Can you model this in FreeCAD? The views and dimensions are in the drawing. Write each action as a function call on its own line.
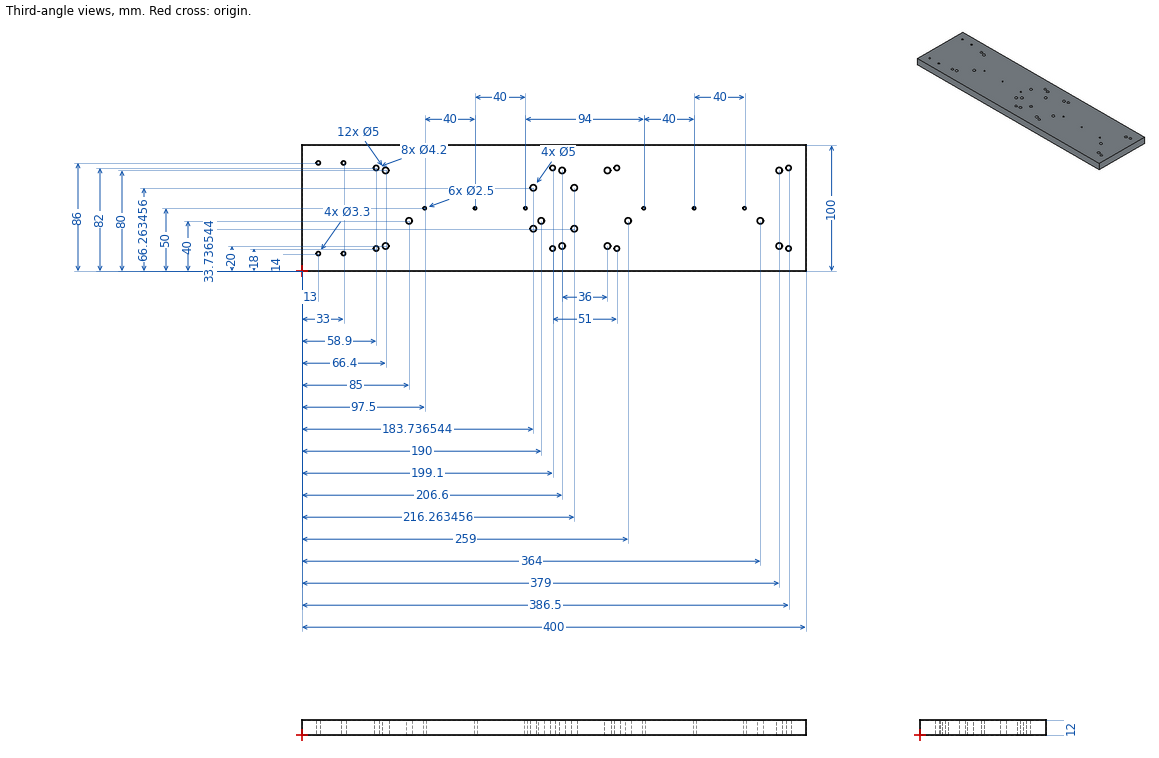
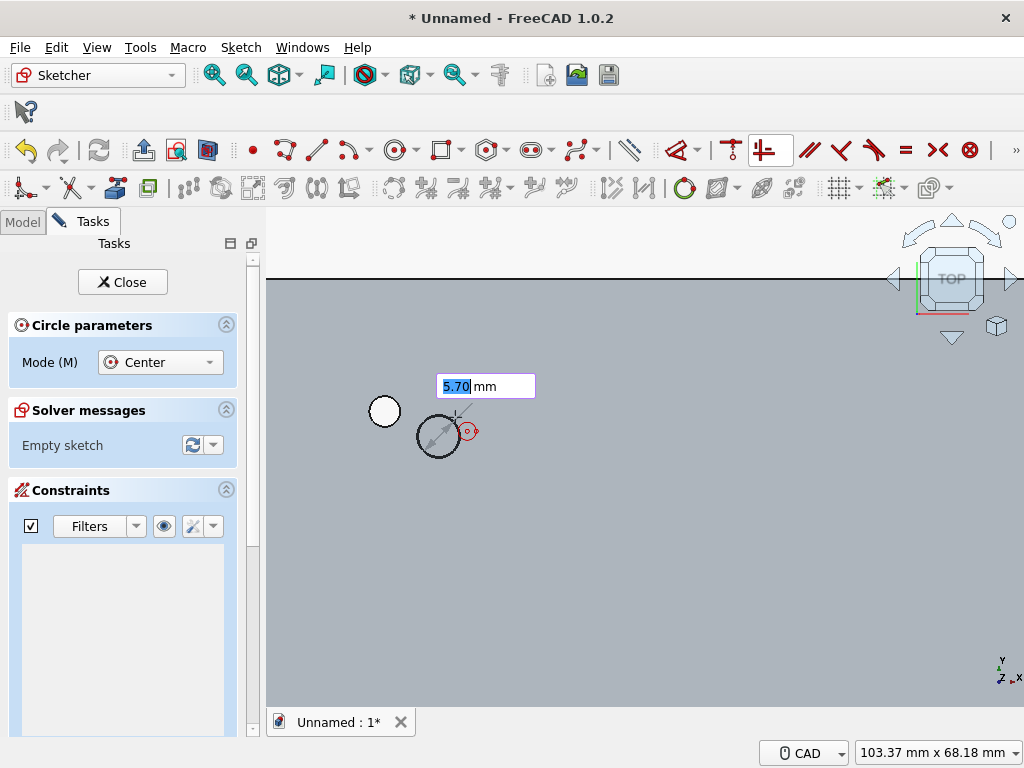
click(453, 413)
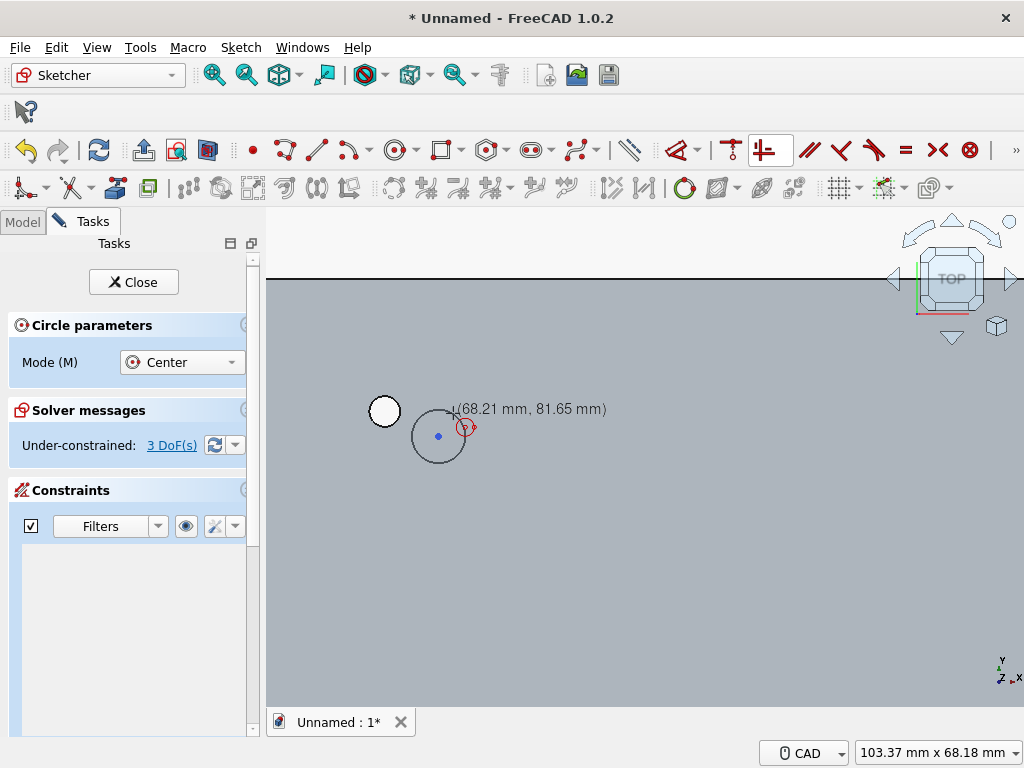
scroll(455, 417, down, 10)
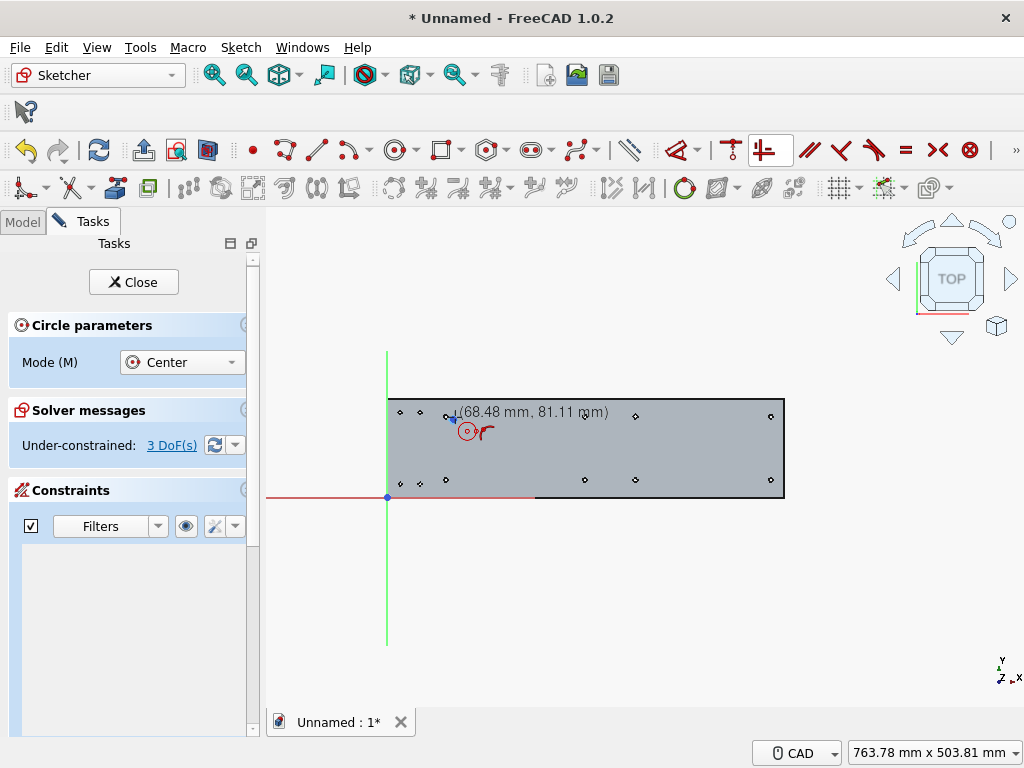
scroll(453, 478, up, 12)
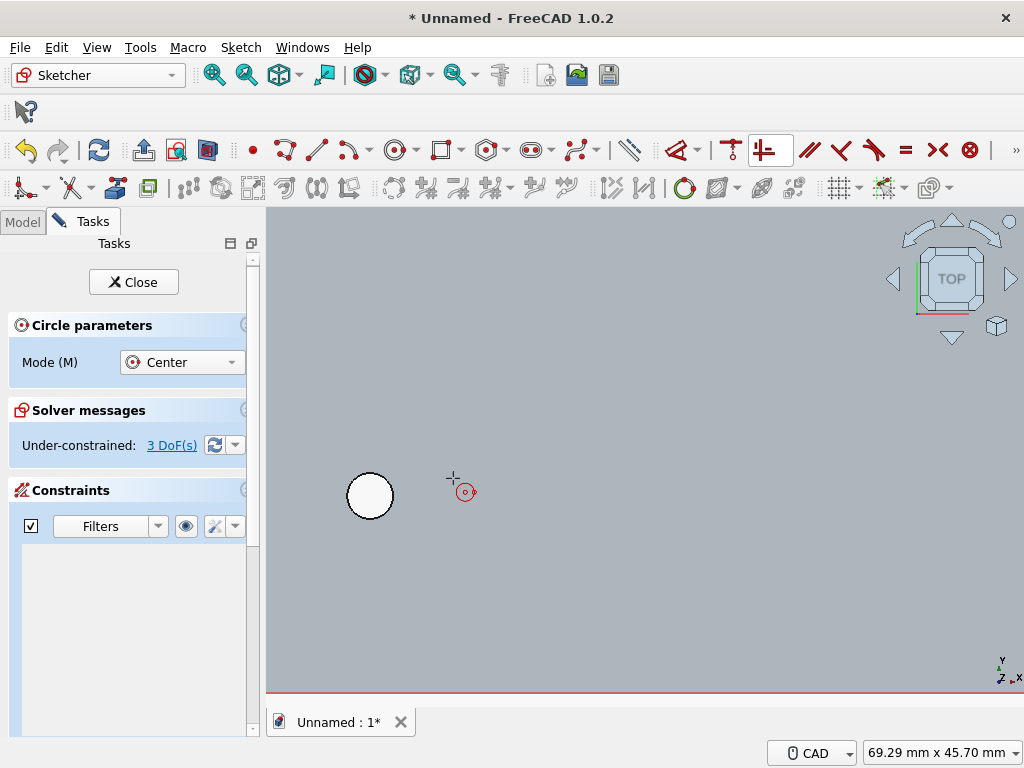
scroll(453, 478, down, 12)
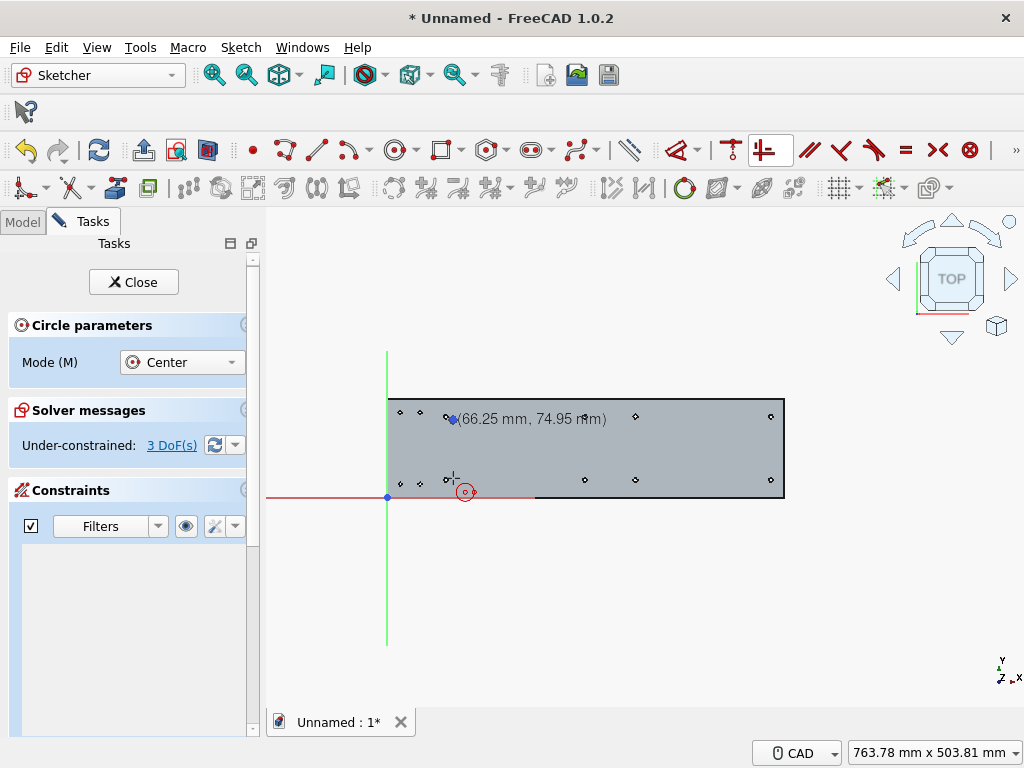
click(453, 478)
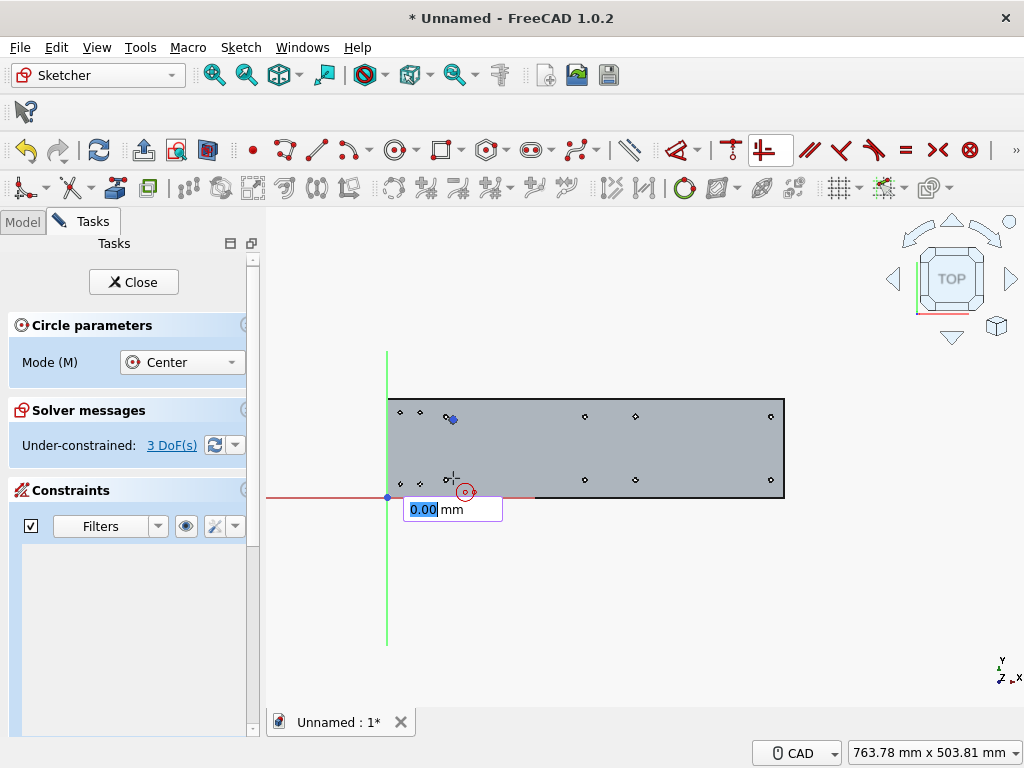
scroll(455, 476, up, 10)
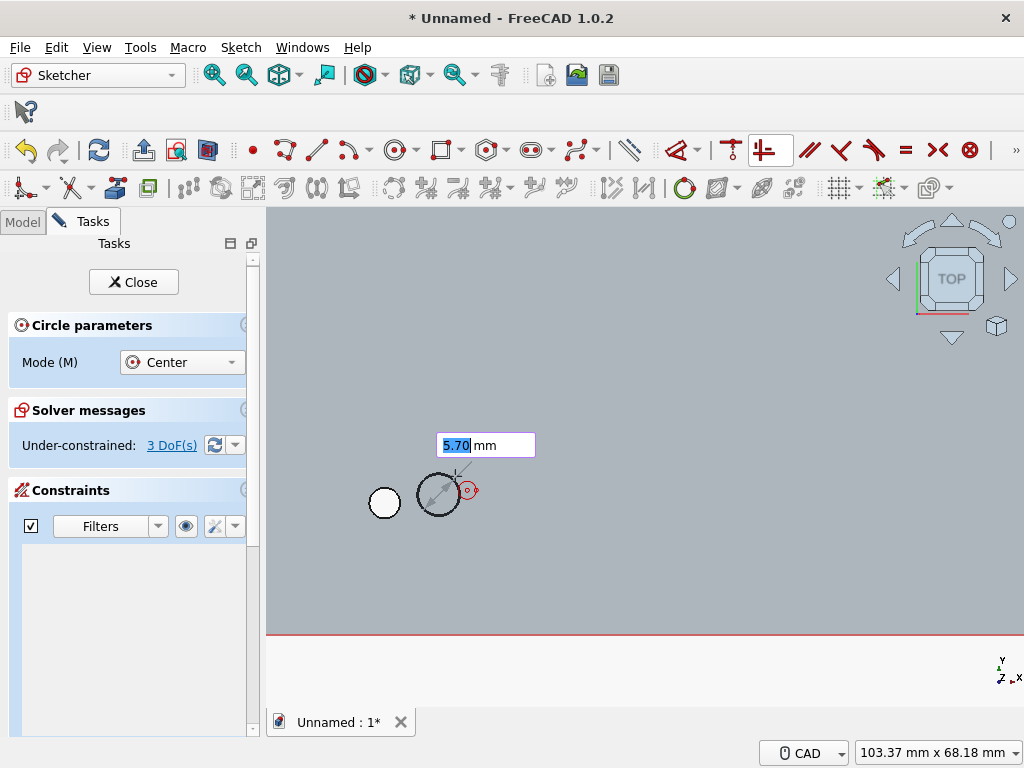
click(453, 475)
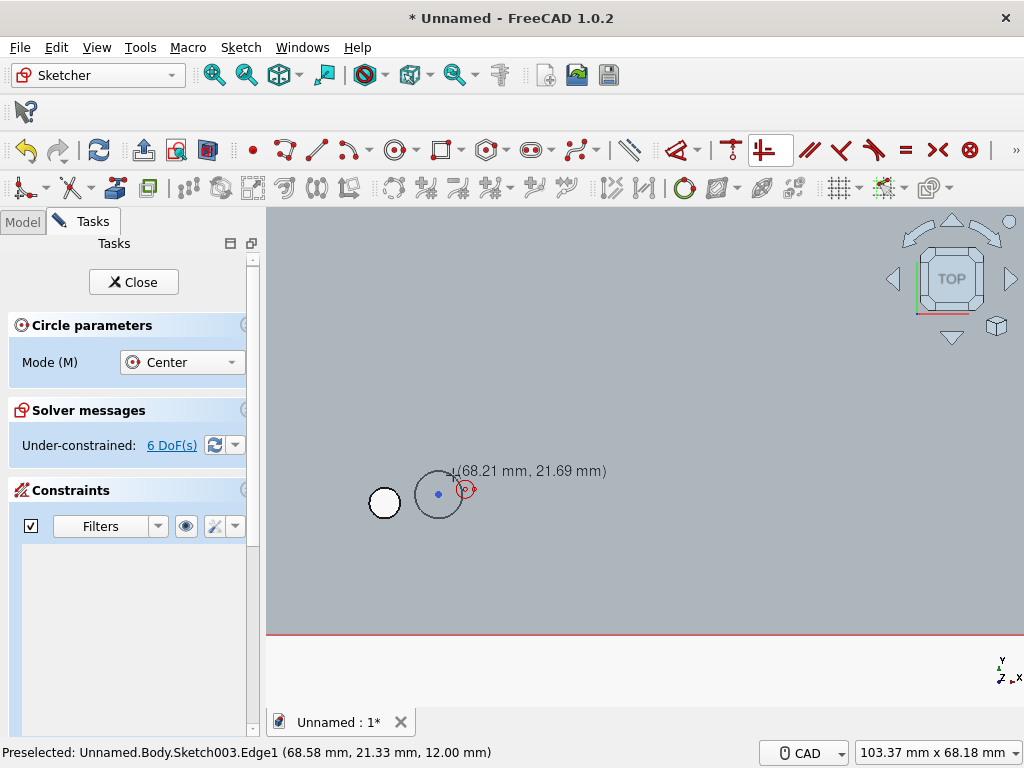
scroll(455, 476, down, 10)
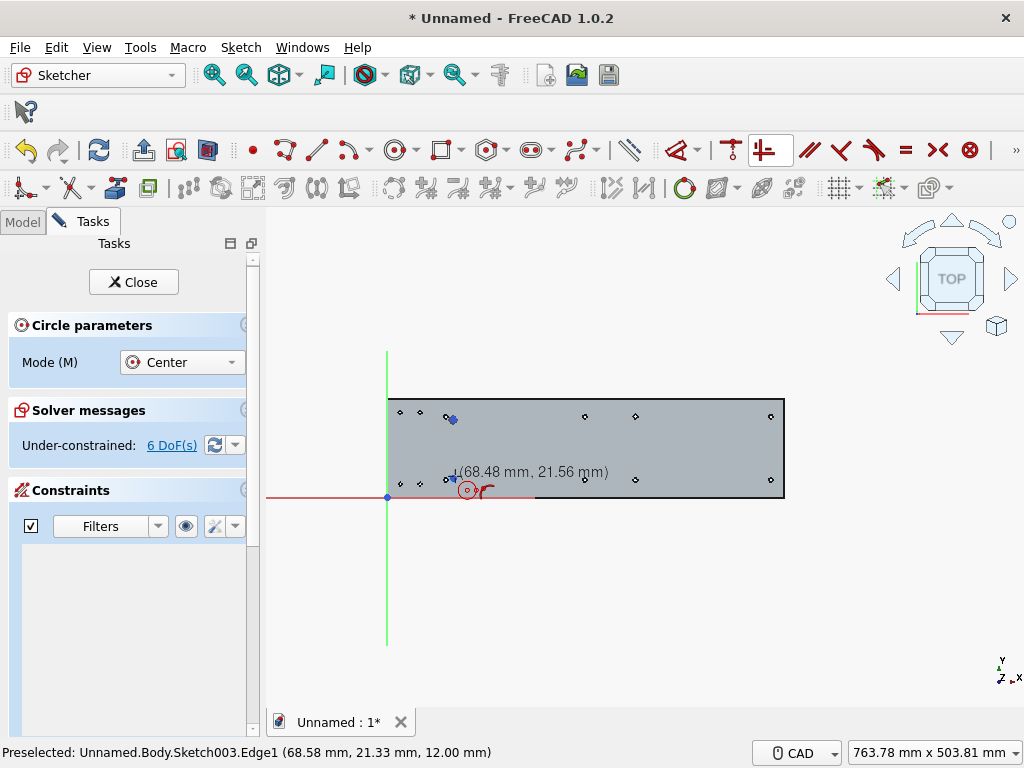
scroll(592, 419, up, 12)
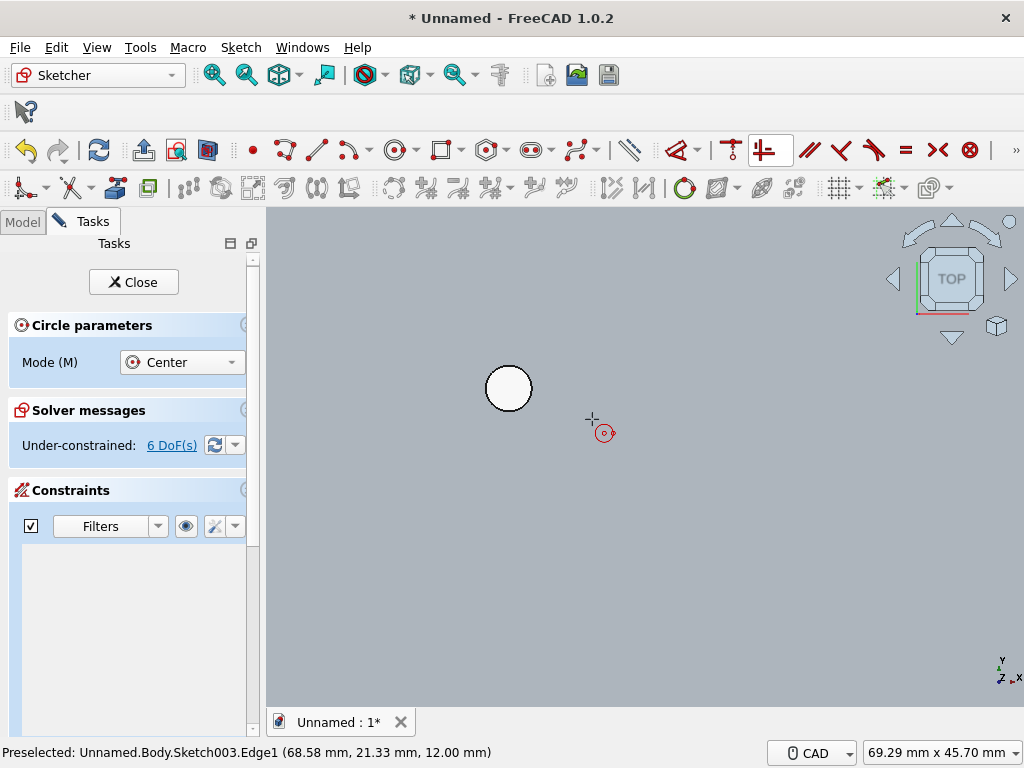
scroll(592, 419, down, 12)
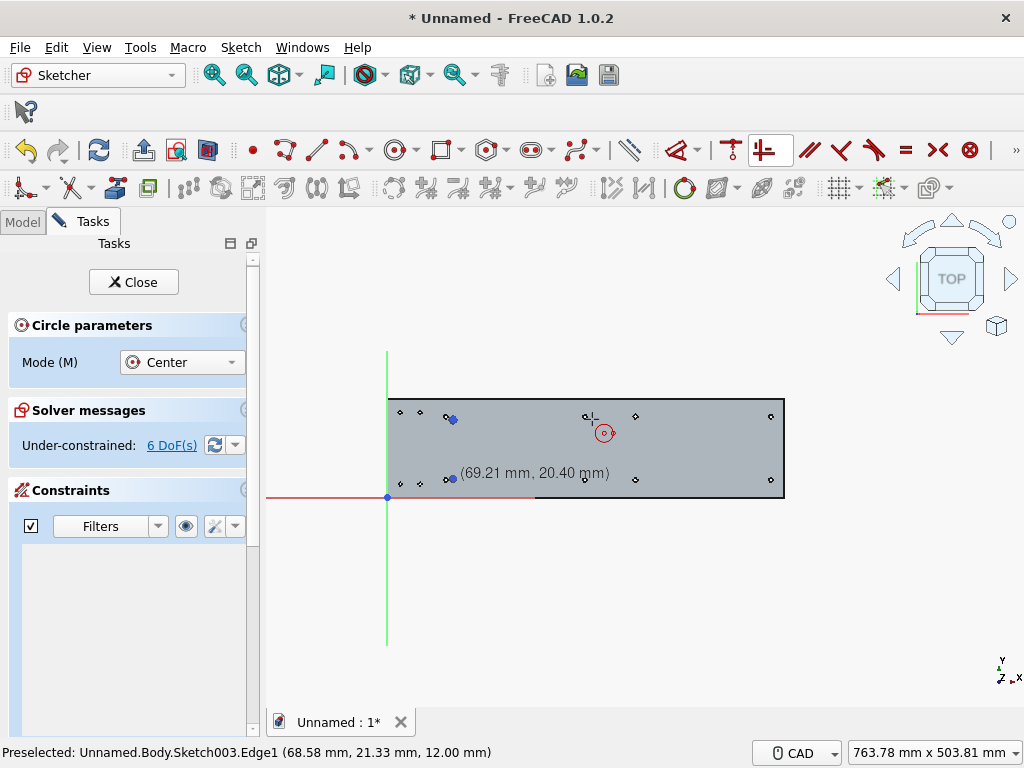
click(592, 419)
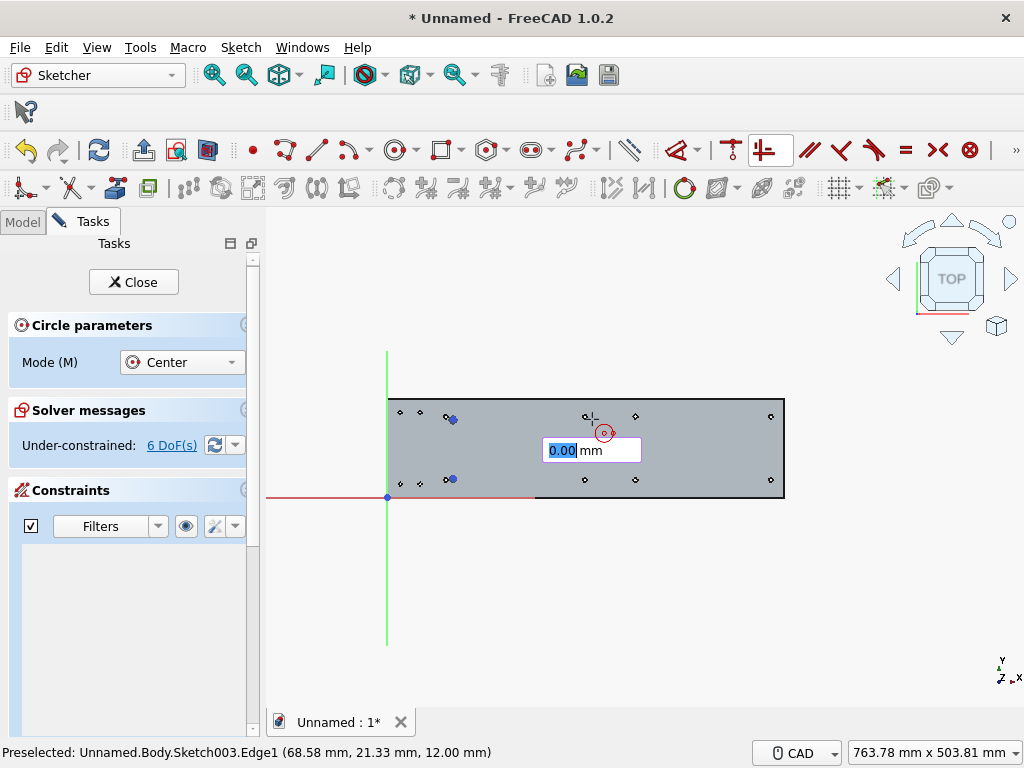
scroll(594, 417, up, 10)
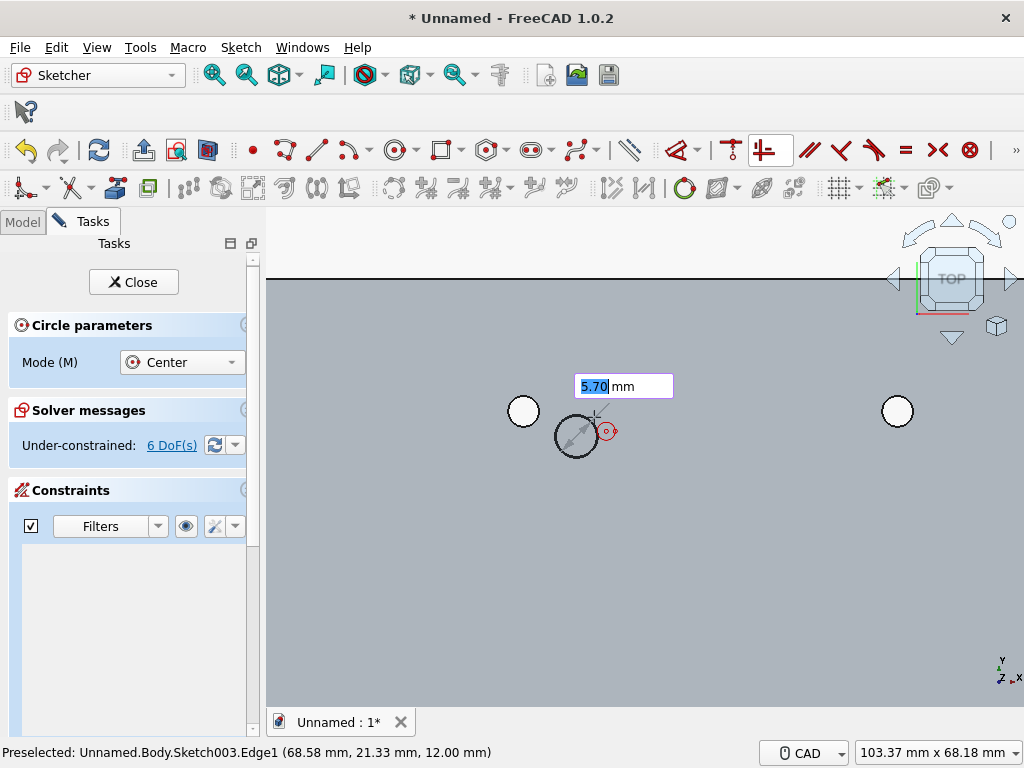
click(592, 413)